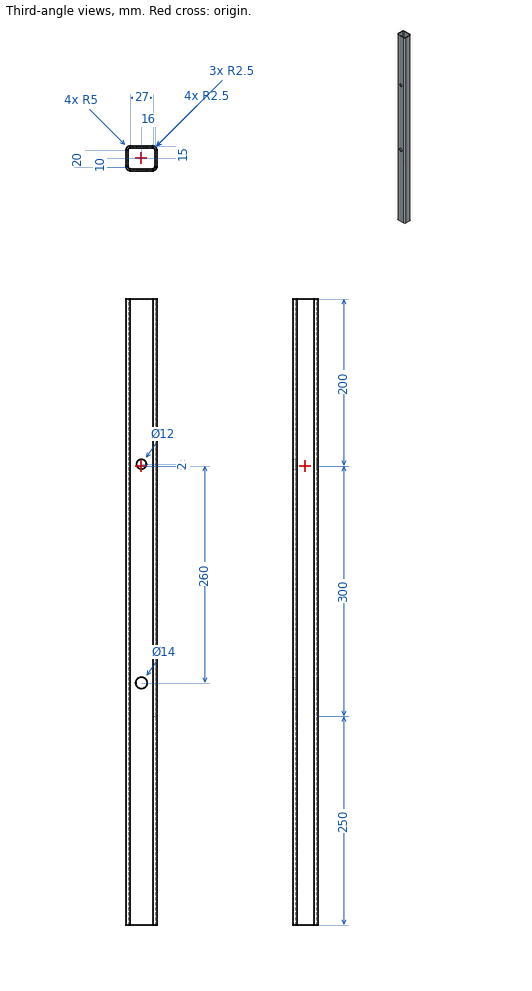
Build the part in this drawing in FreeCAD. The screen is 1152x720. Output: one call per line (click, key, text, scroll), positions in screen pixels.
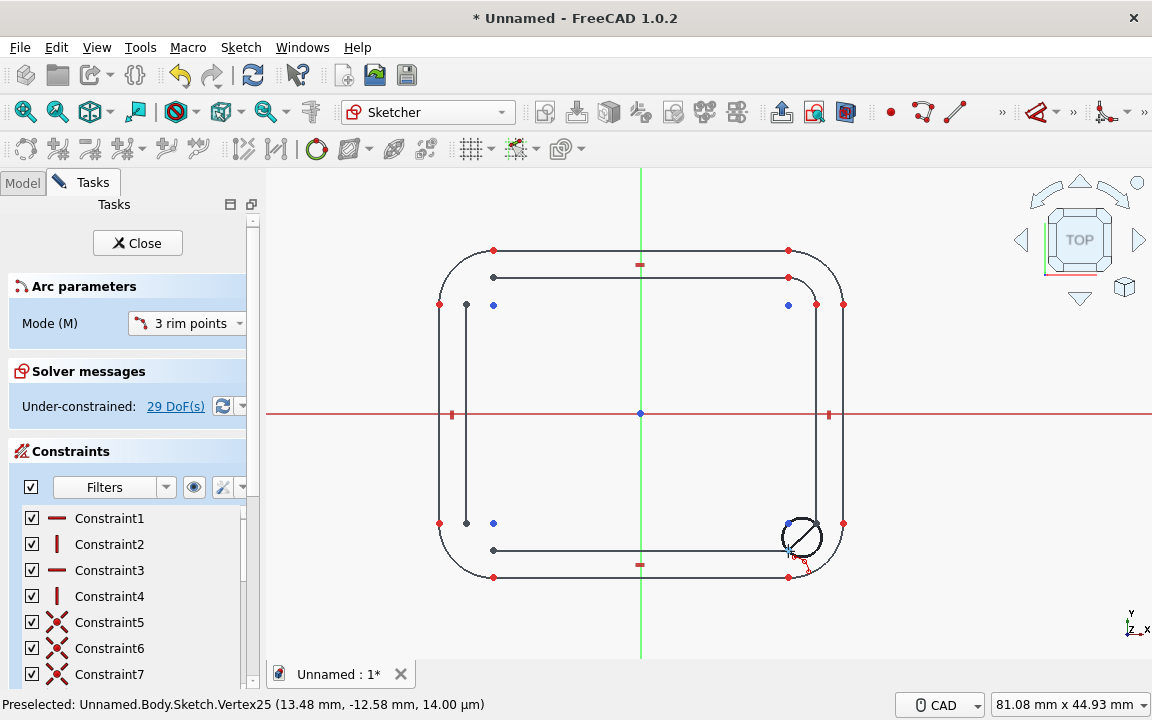
scroll(808, 542, up, 4)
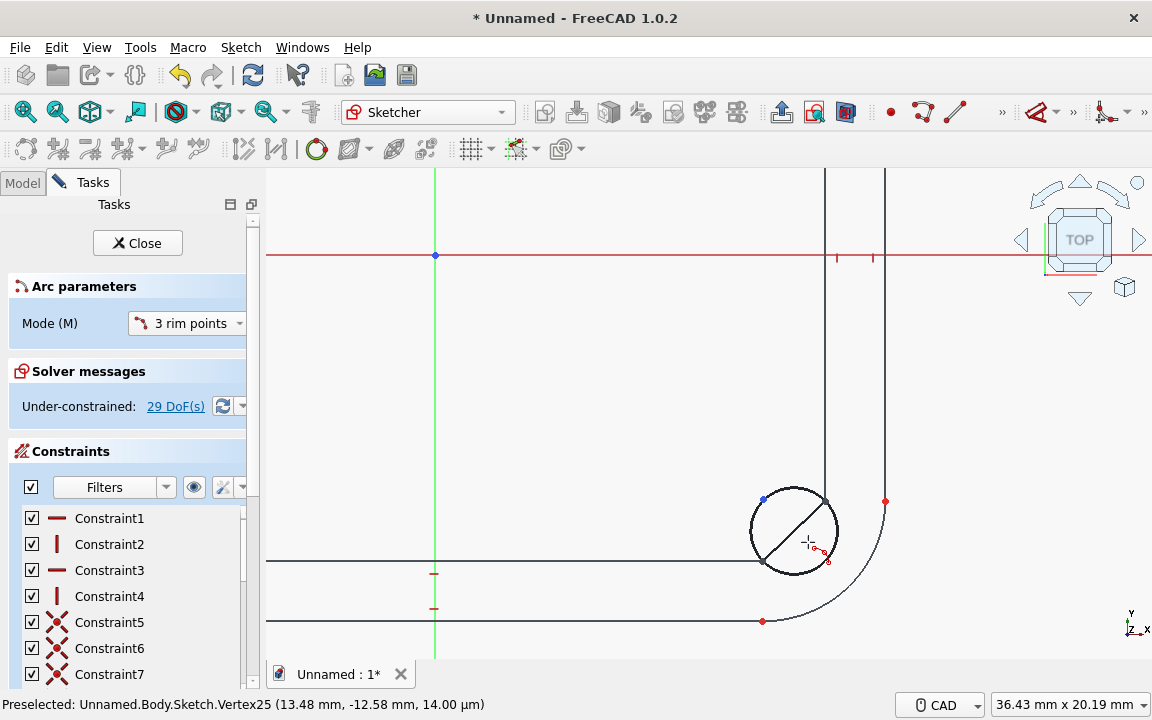
click(806, 541)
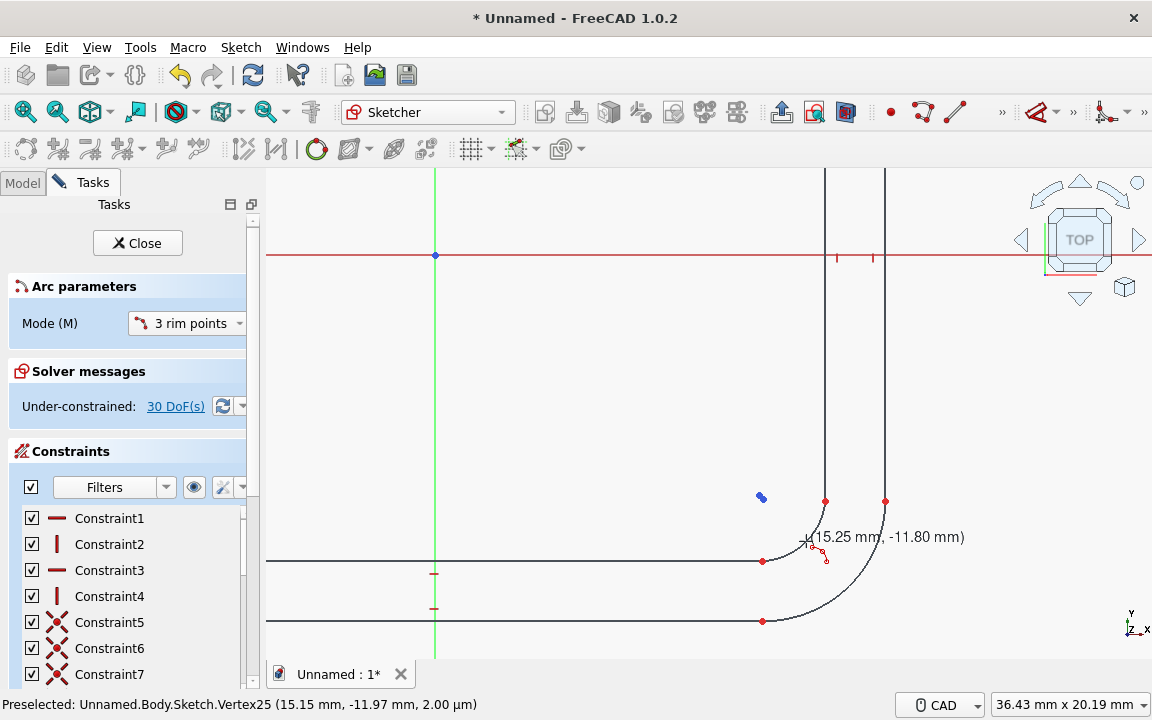
scroll(808, 543, down, 4)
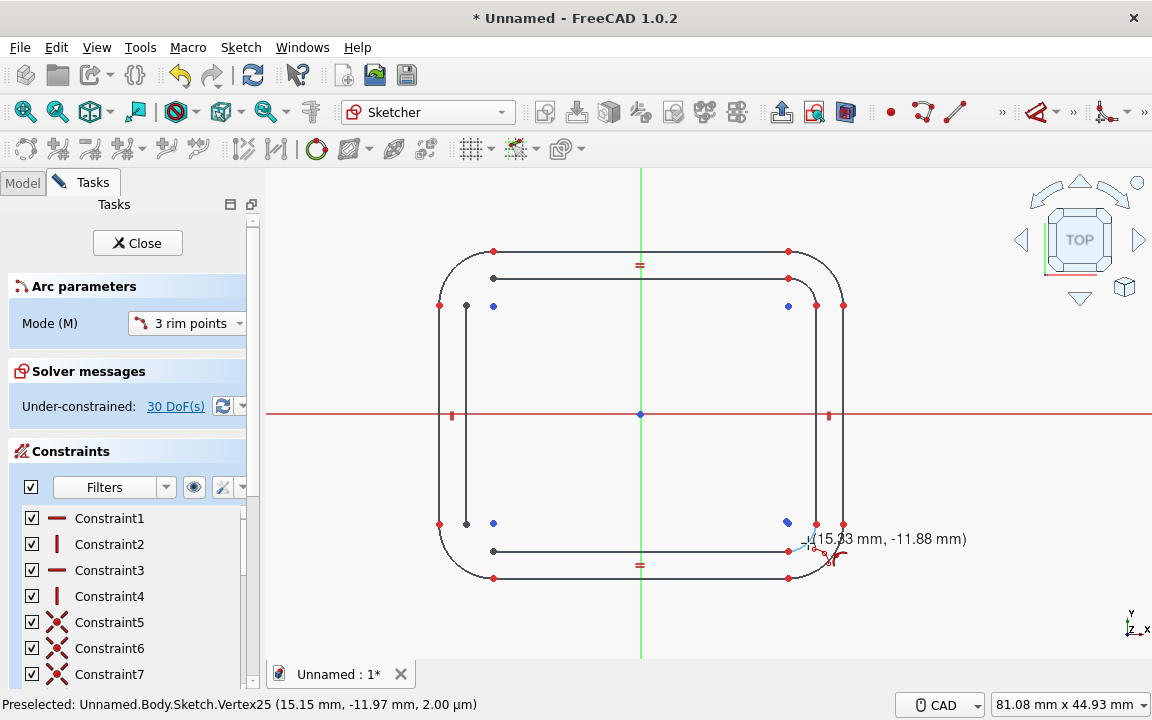
click(493, 552)
click(466, 525)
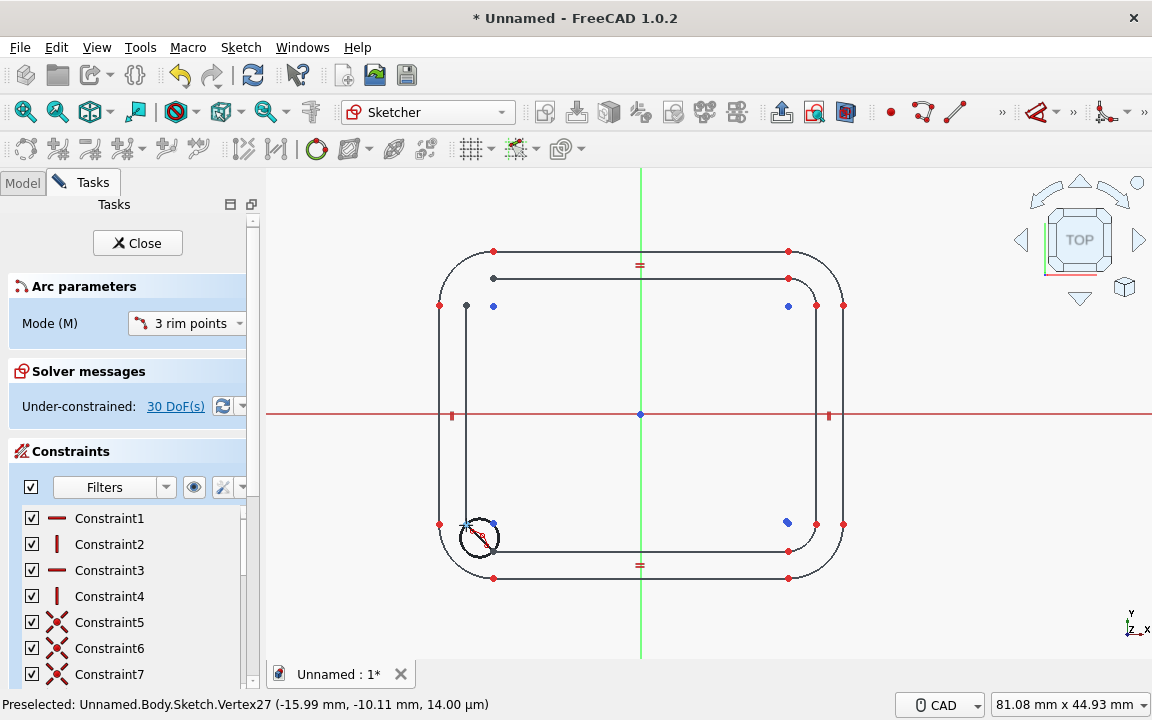
scroll(474, 543, up, 4)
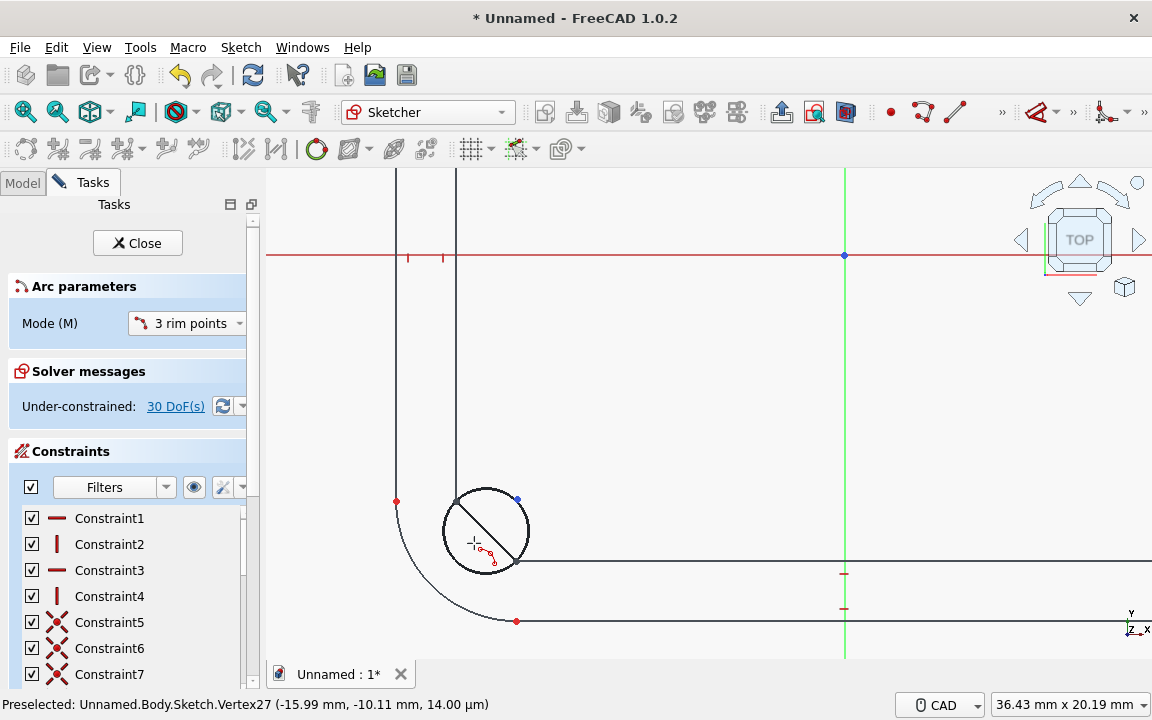
click(474, 541)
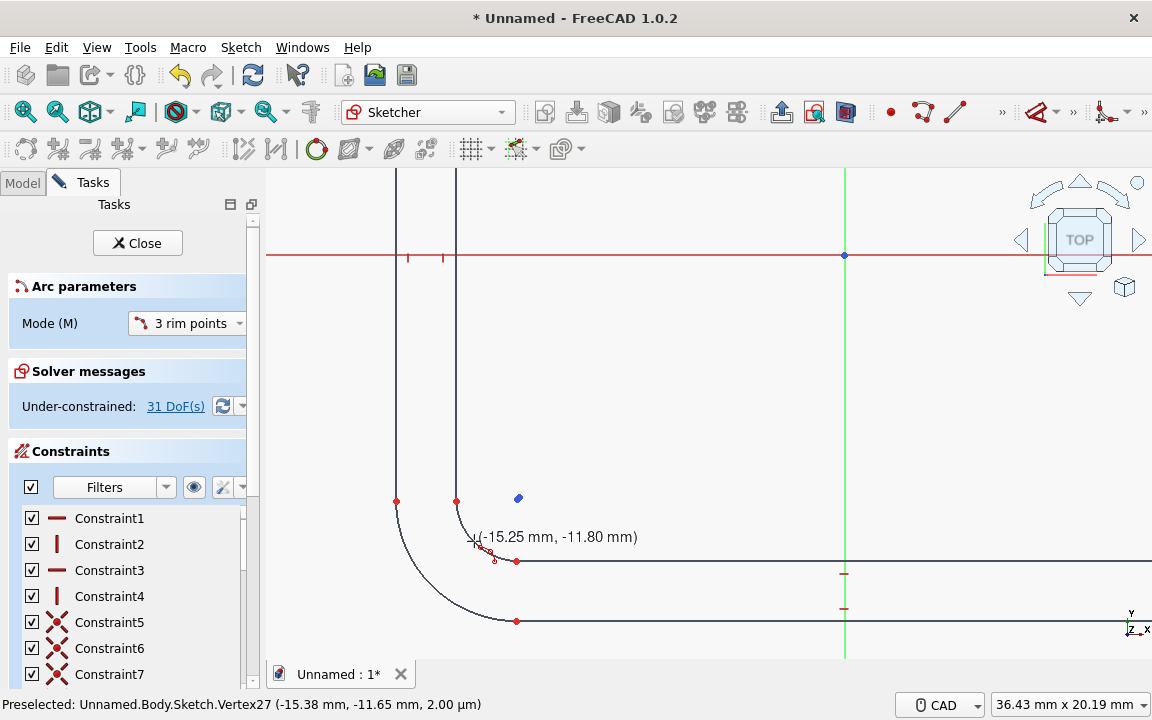
scroll(474, 543, down, 4)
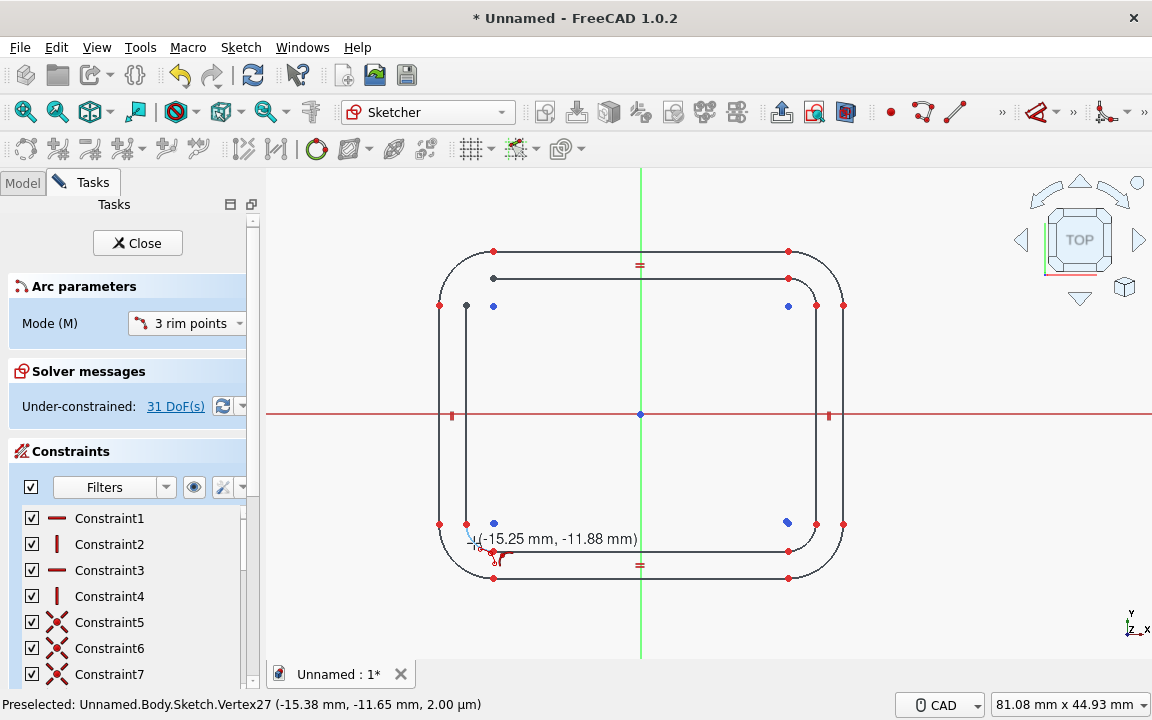
click(466, 306)
click(493, 279)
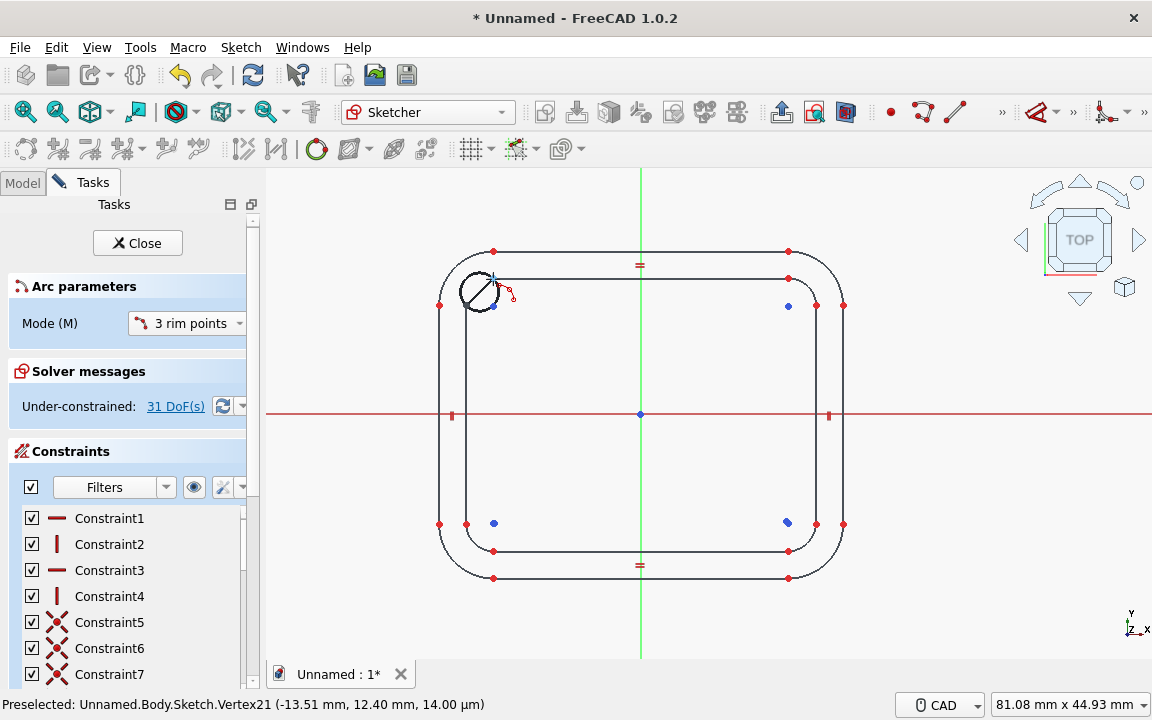
scroll(474, 285, up, 4)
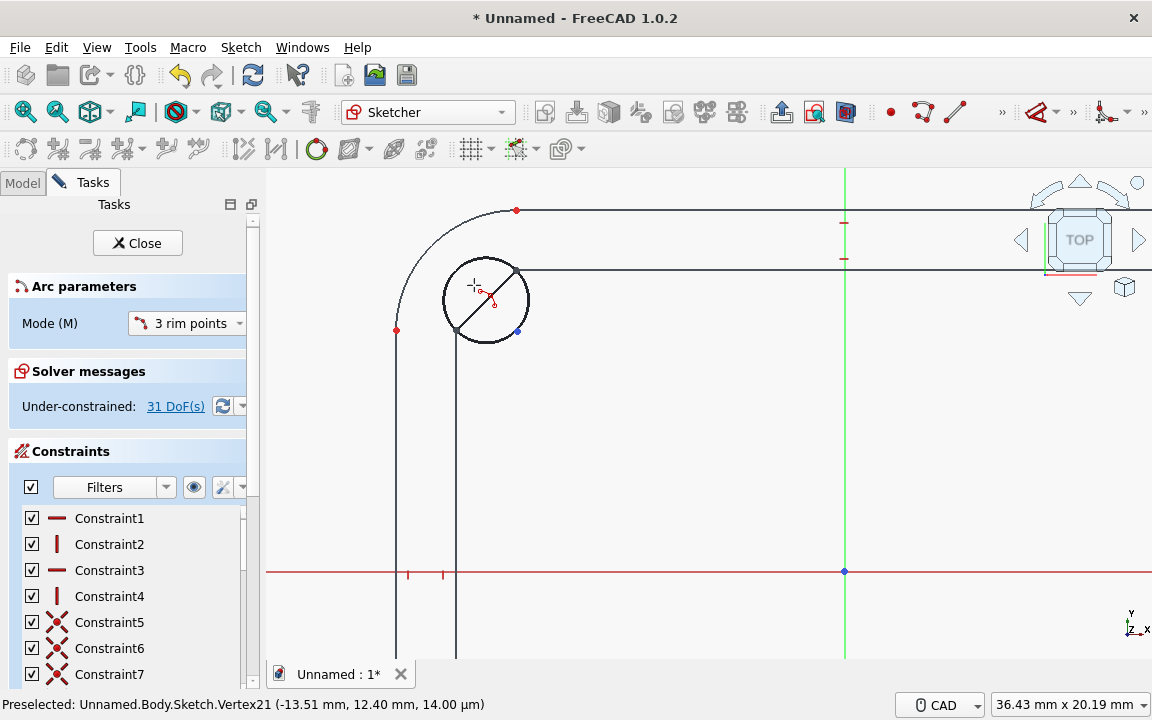
click(474, 286)
key(Escape)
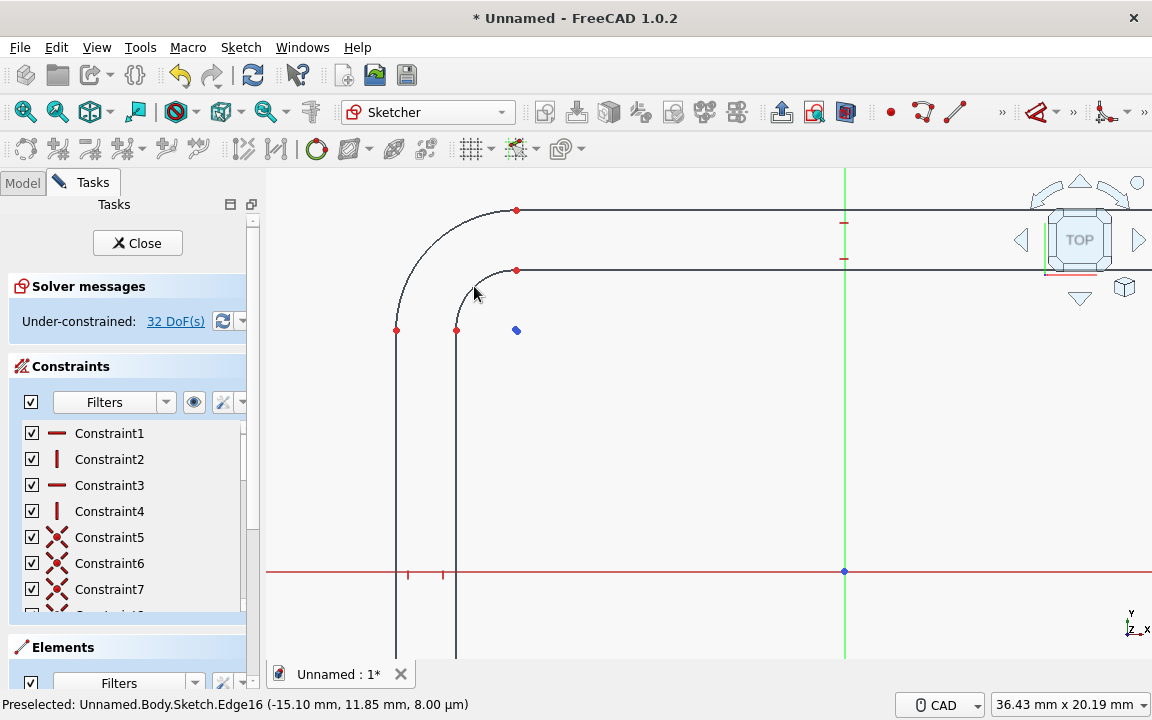
click(976, 210)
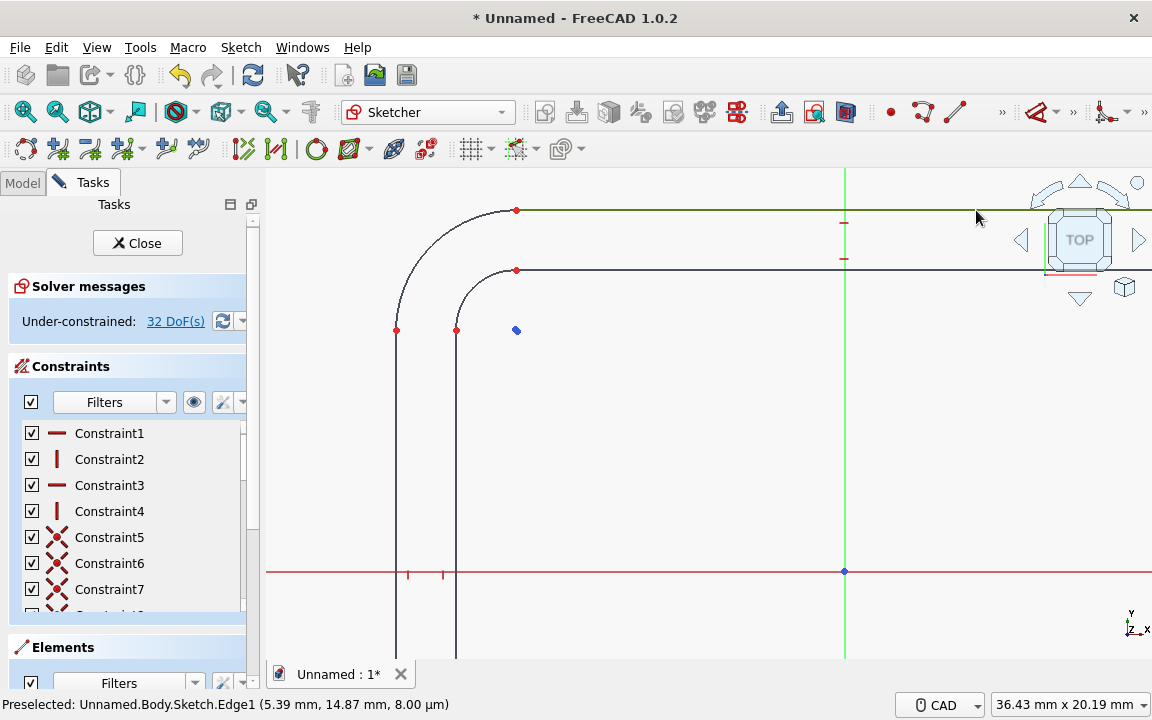
click(462, 224)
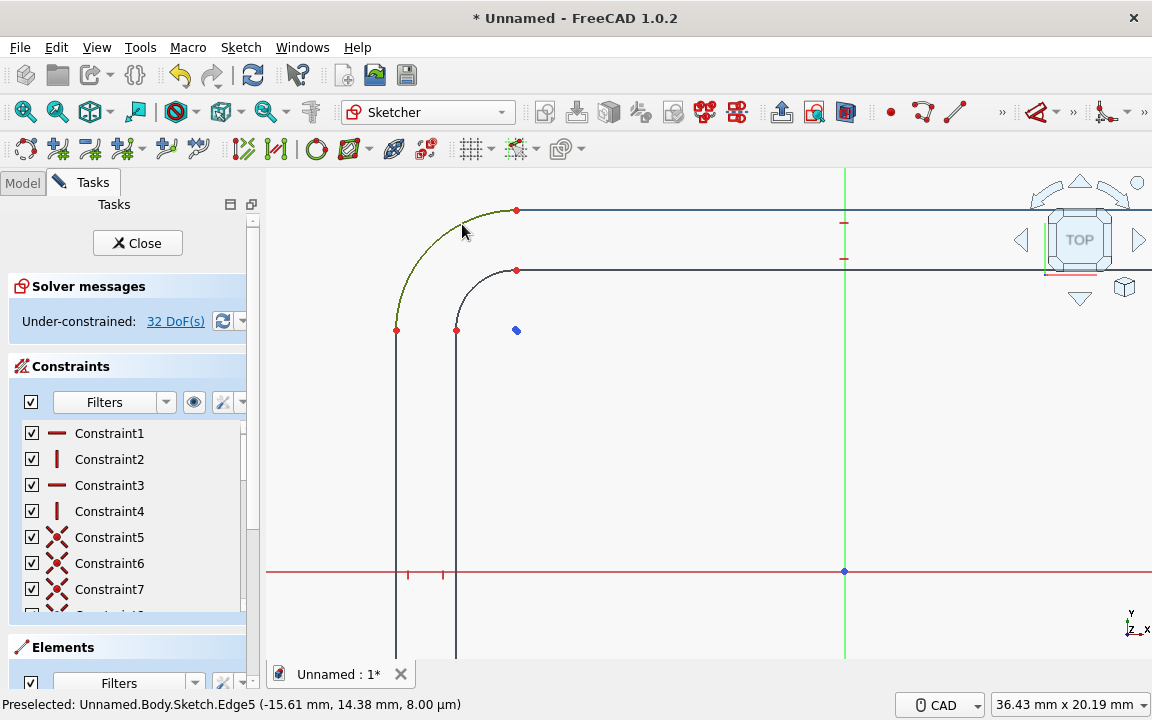
key(t)